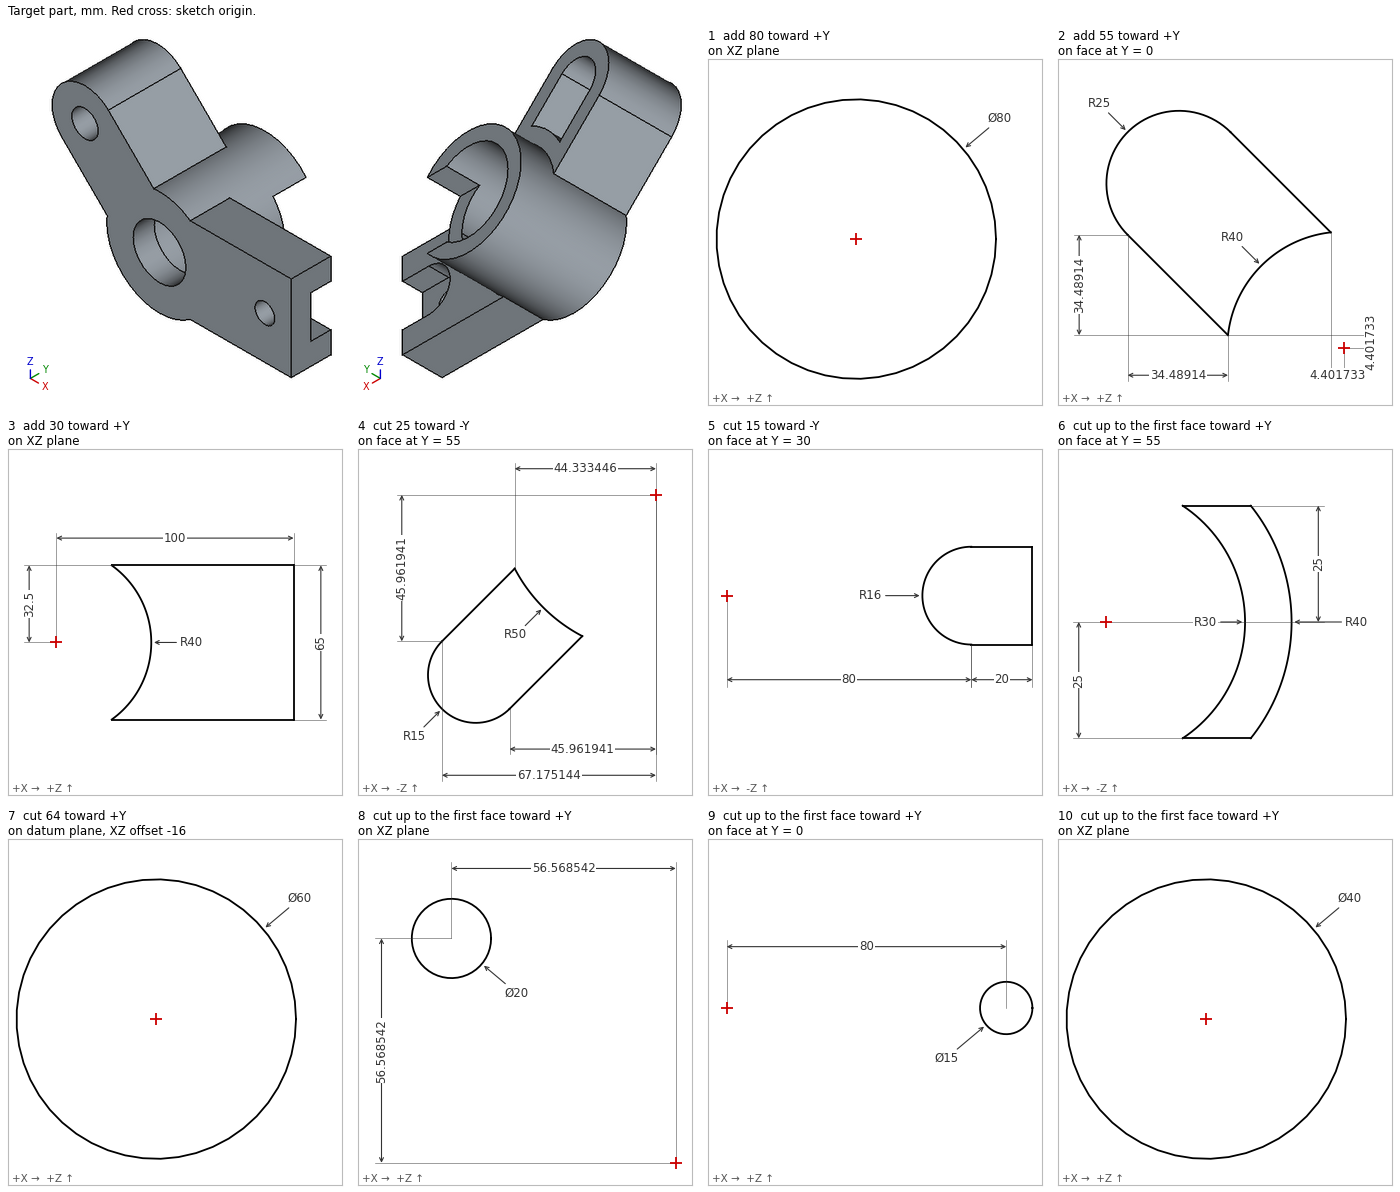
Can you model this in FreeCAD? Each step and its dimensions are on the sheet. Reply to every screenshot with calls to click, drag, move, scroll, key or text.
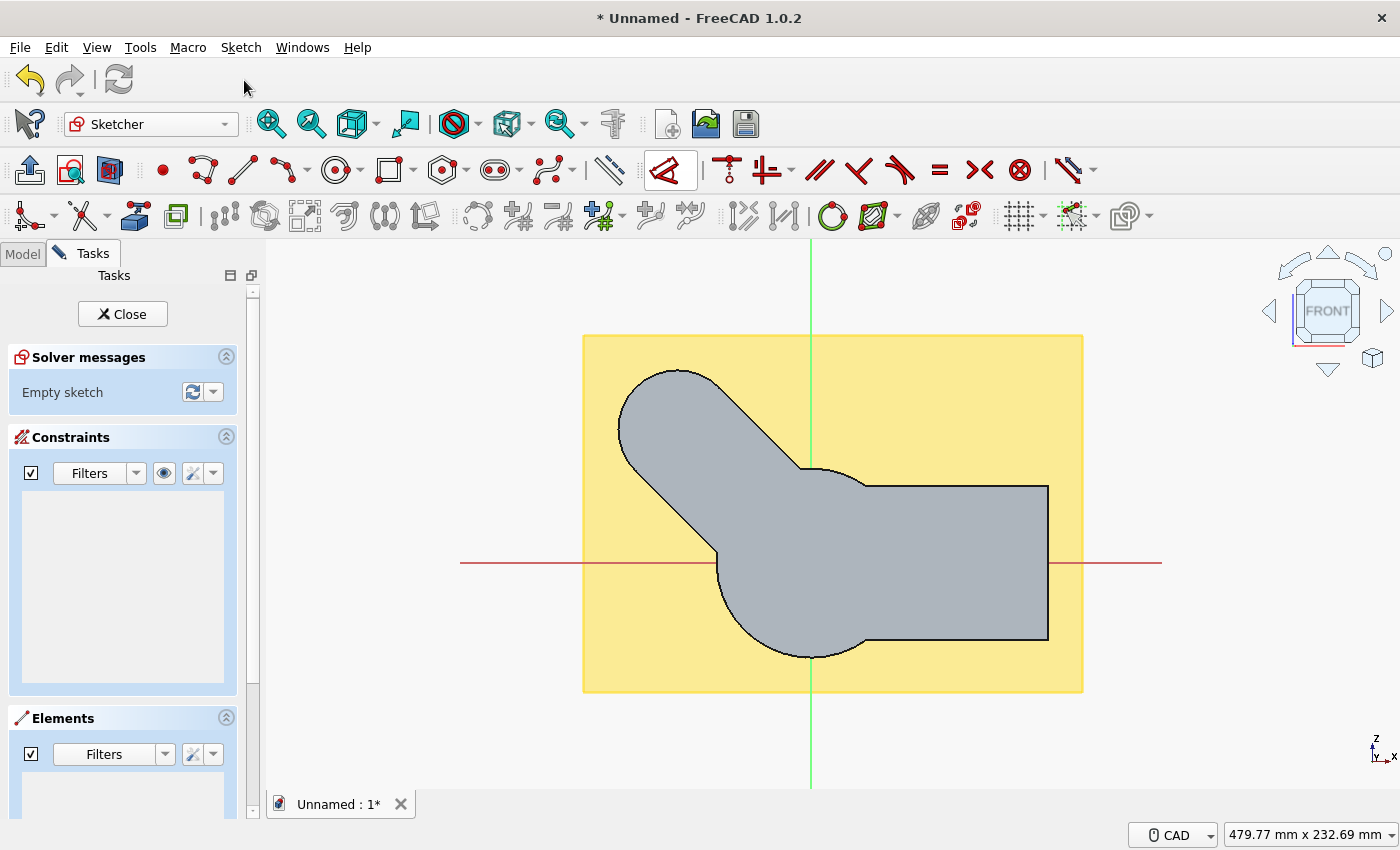
click(110, 170)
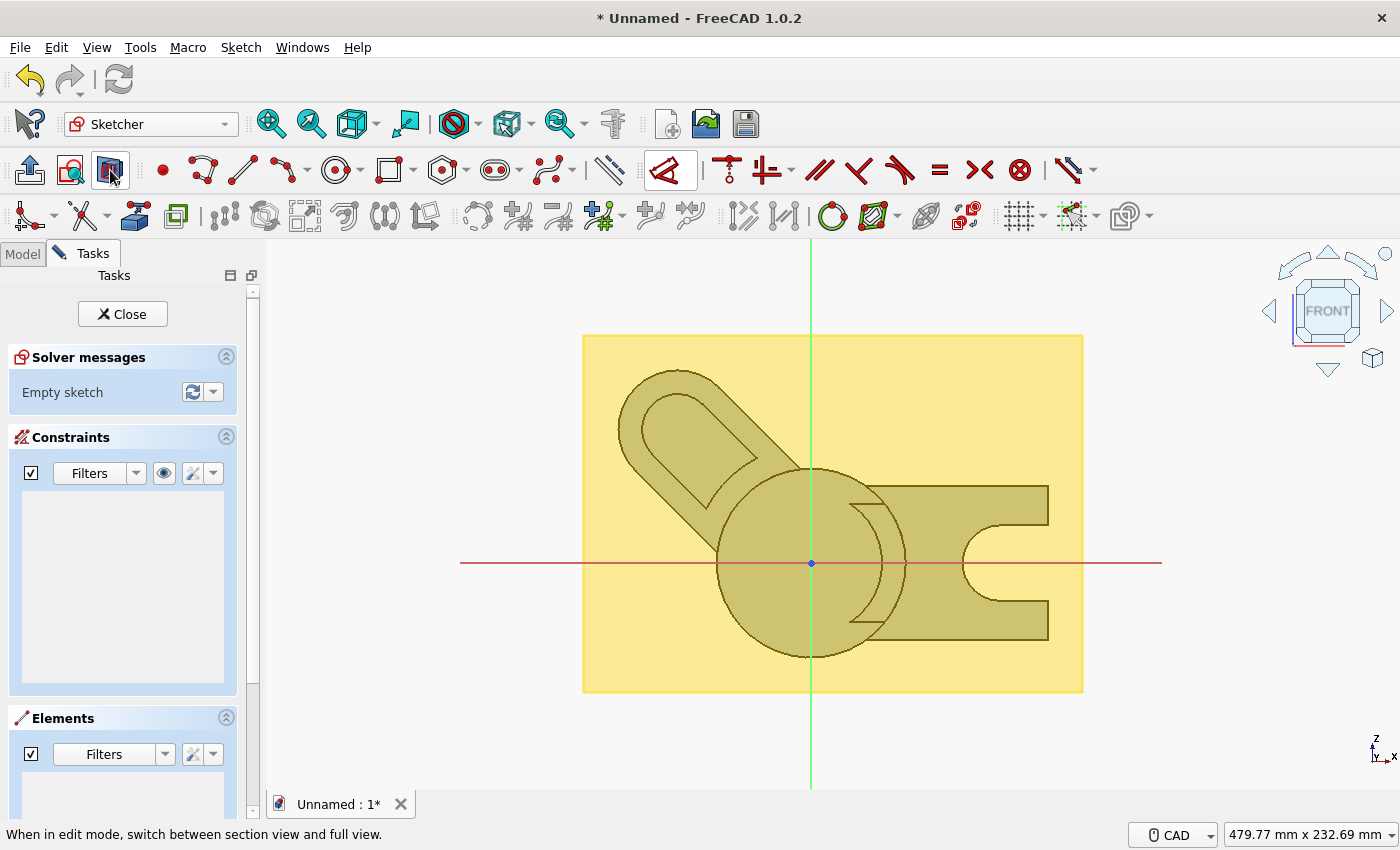
scroll(849, 603, up, 4)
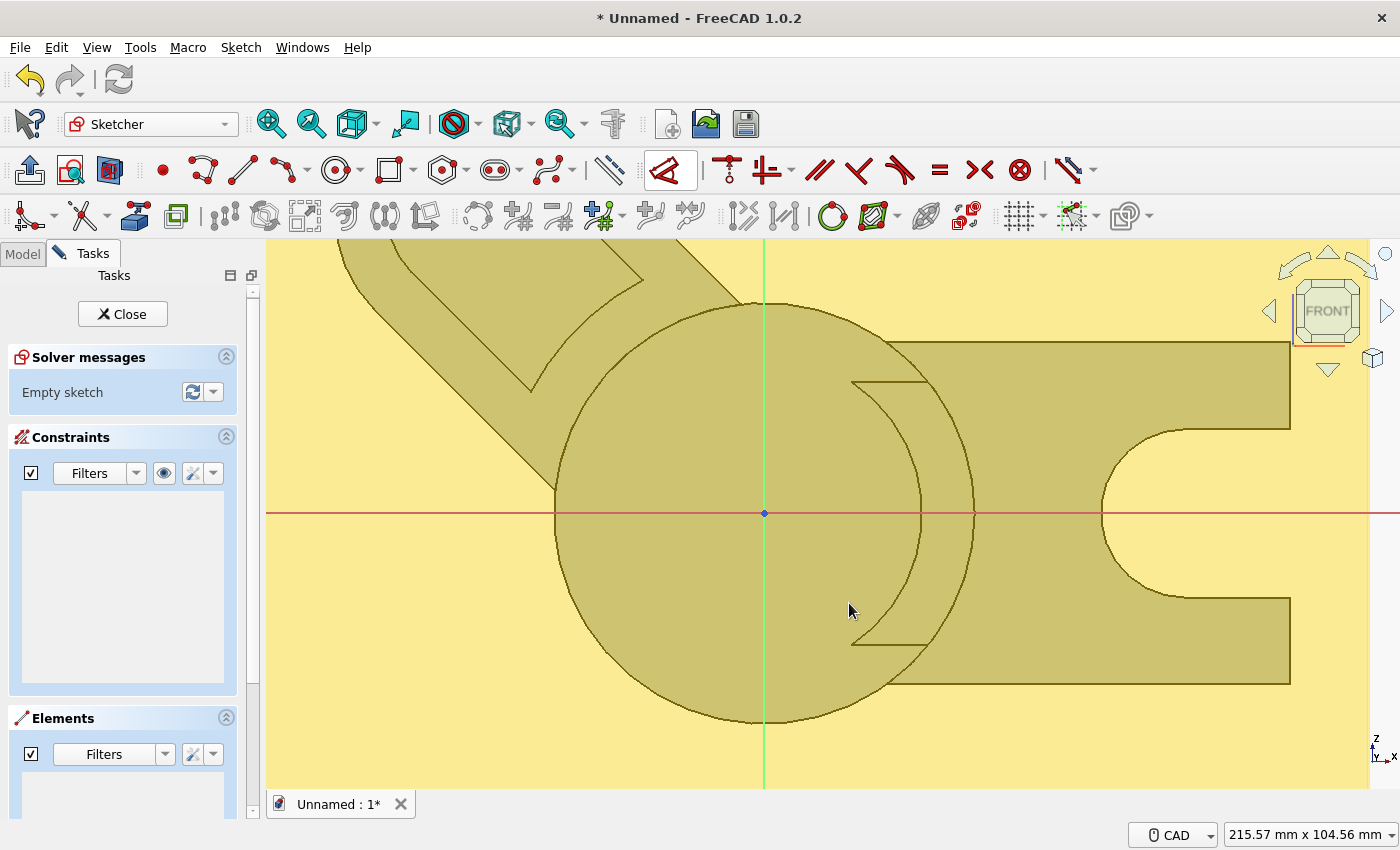
click(336, 170)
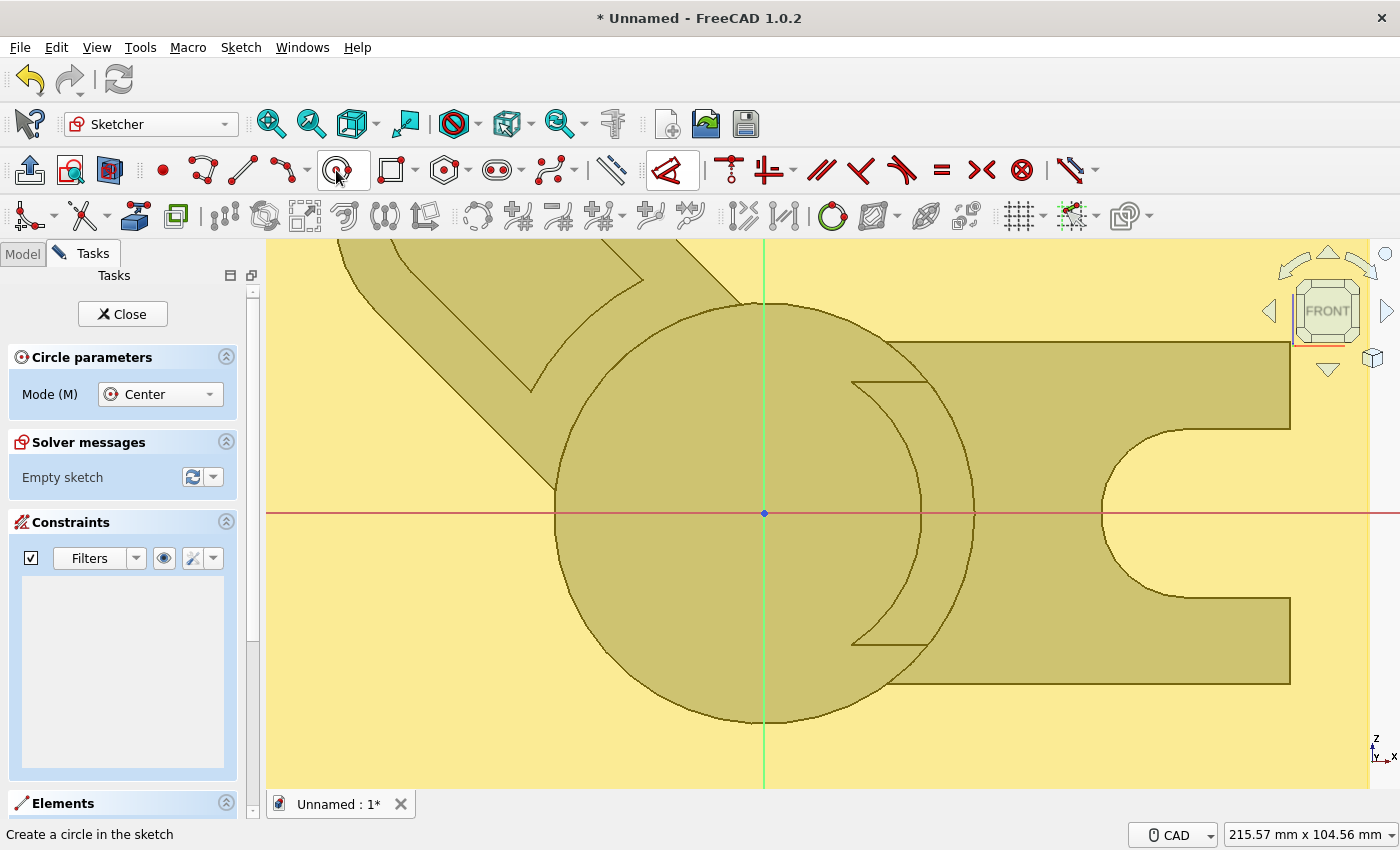
click(764, 513)
click(876, 402)
key(Escape)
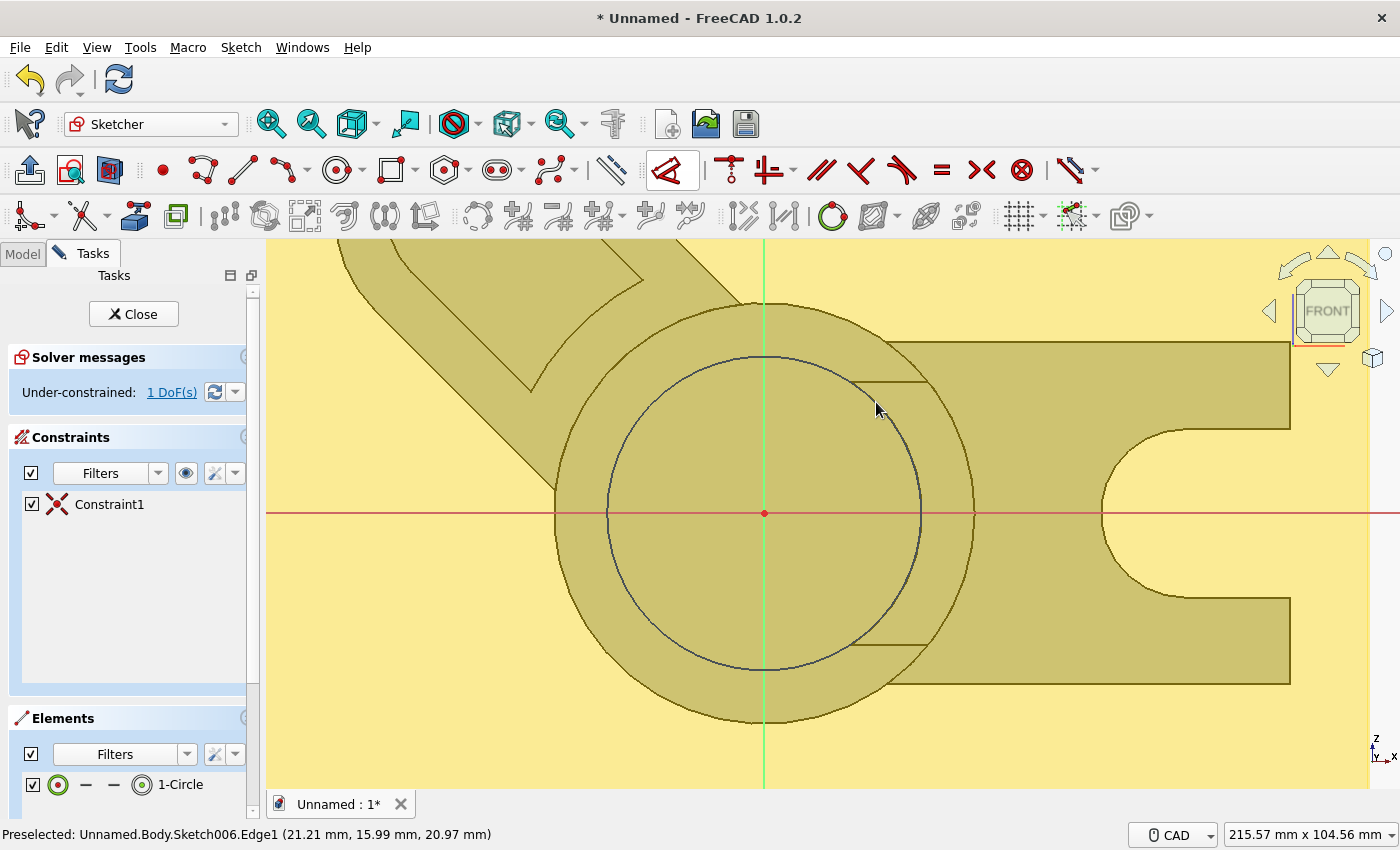
click(875, 402)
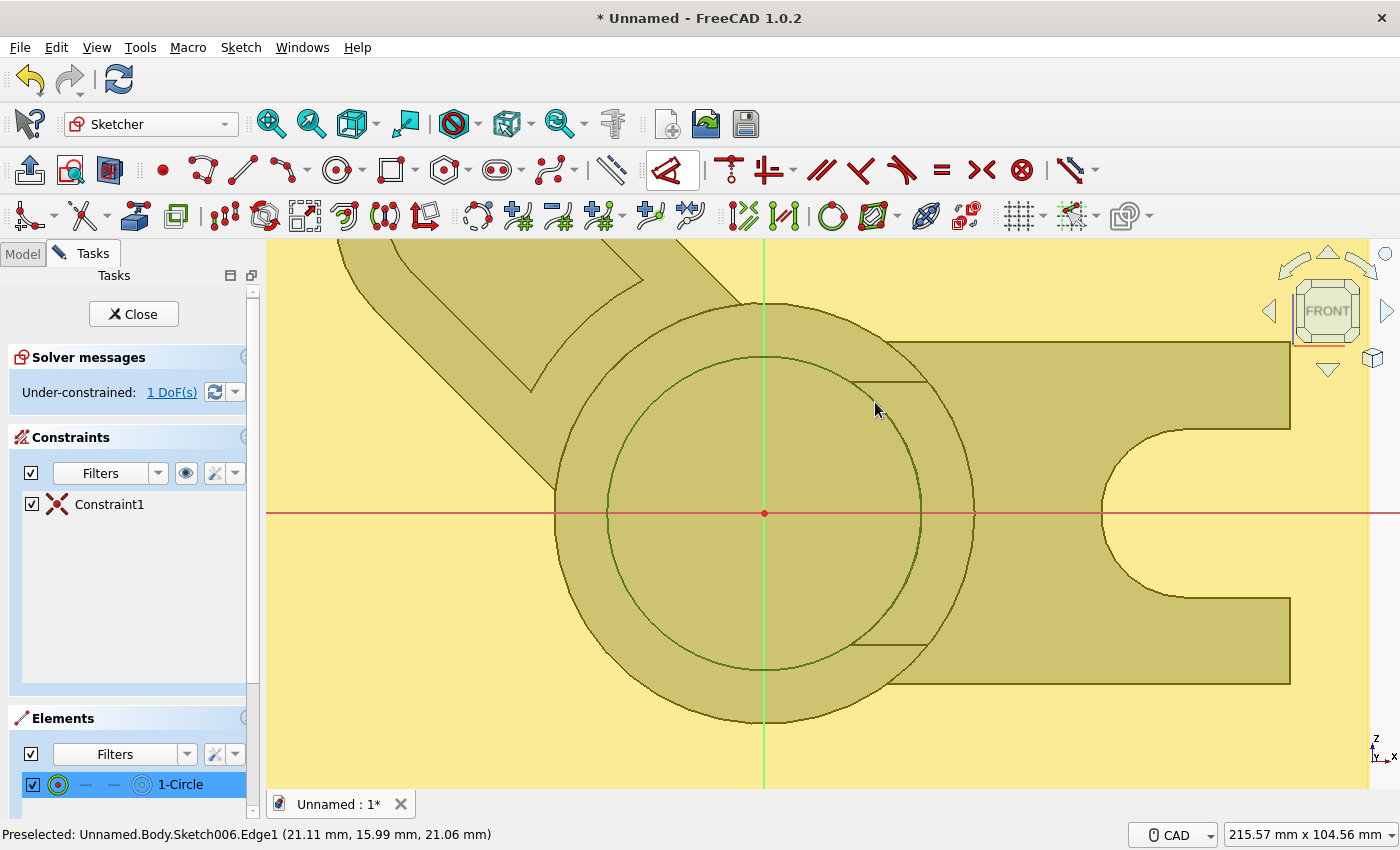
click(694, 170)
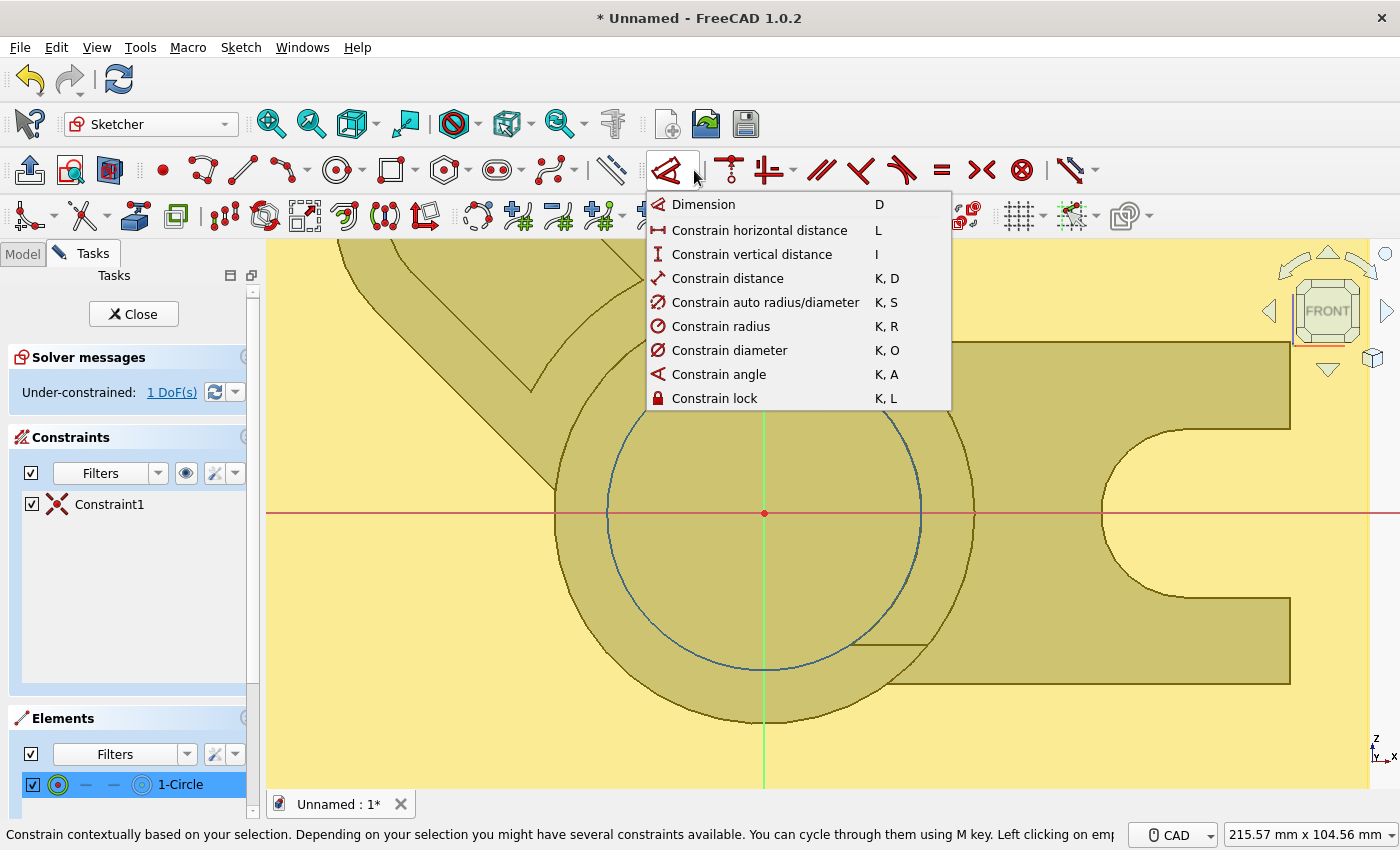
click(799, 350)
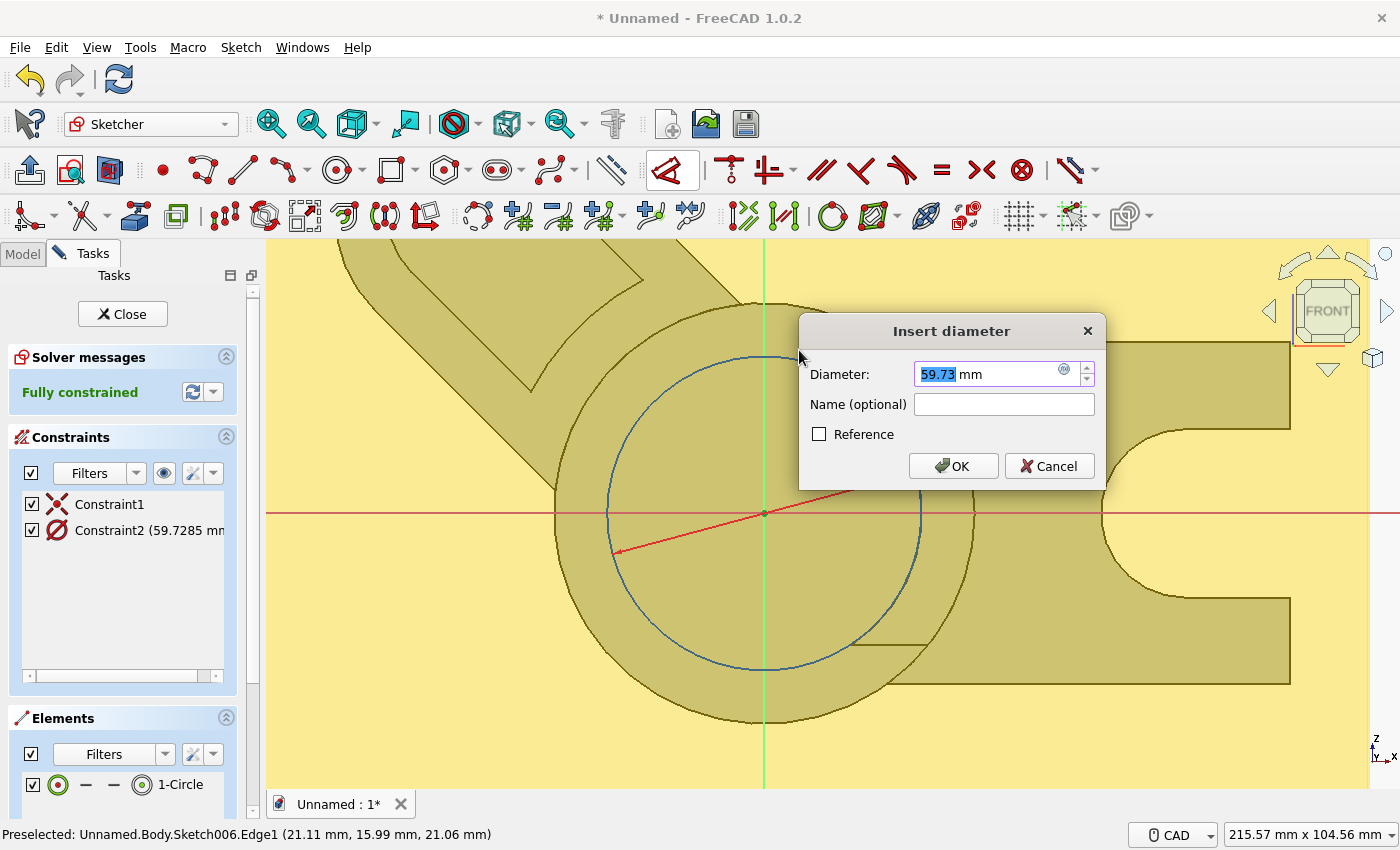
text(60)
key(Return)